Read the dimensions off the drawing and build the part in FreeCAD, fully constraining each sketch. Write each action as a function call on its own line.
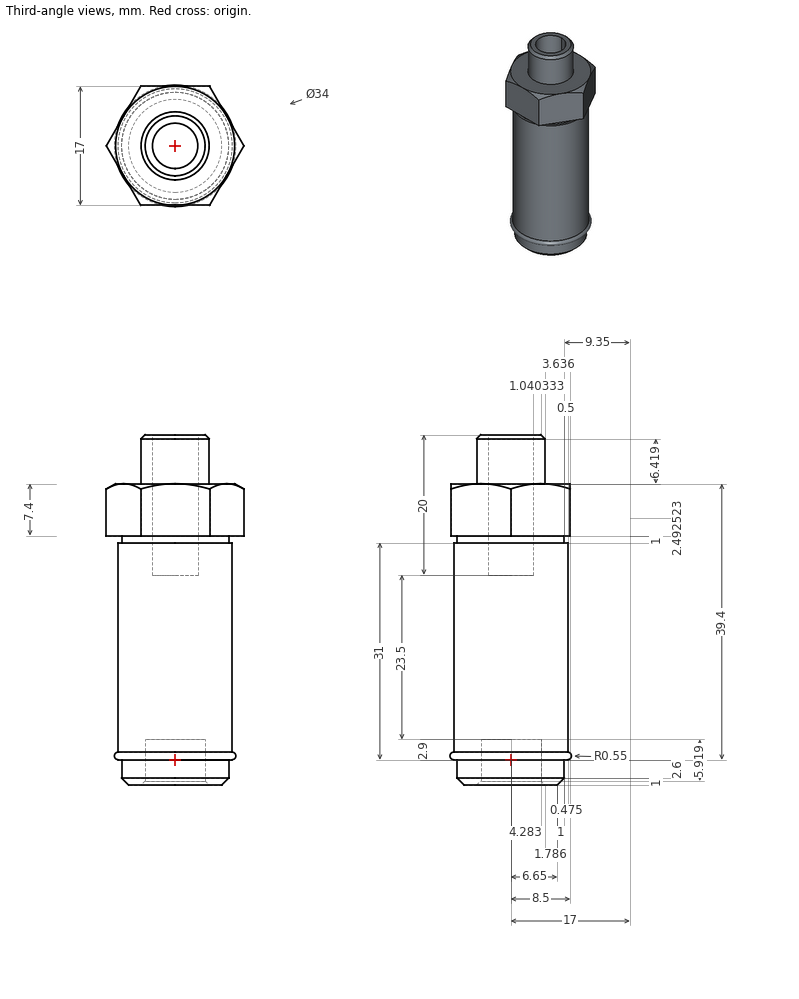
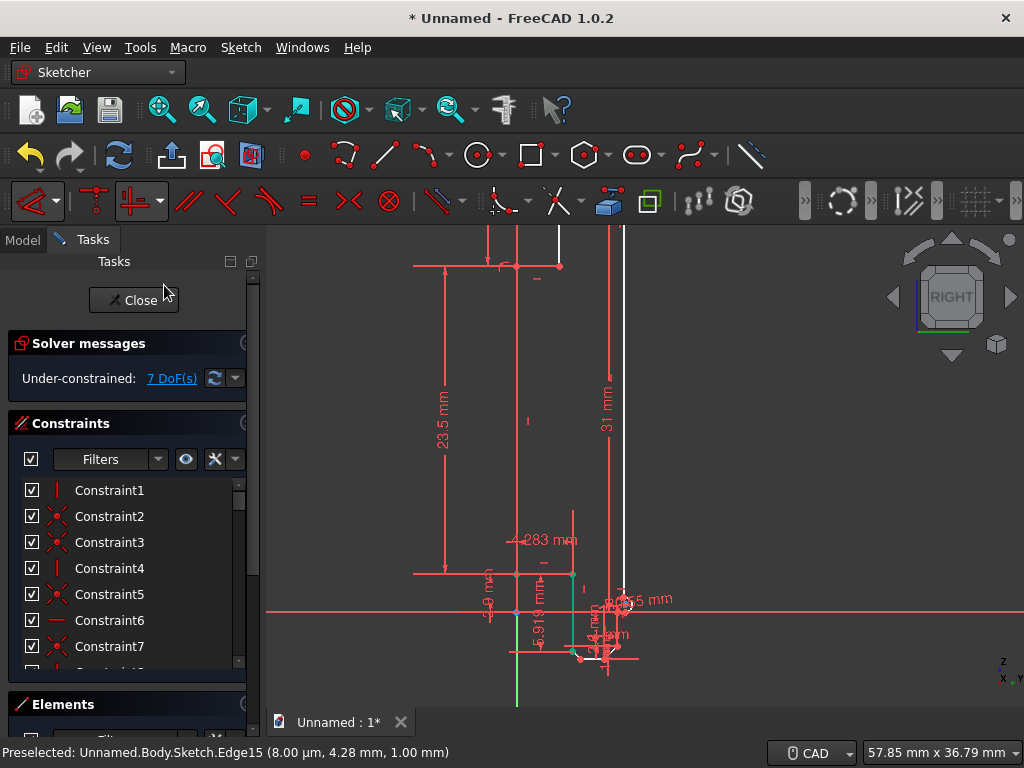
scroll(590, 659, up, 3)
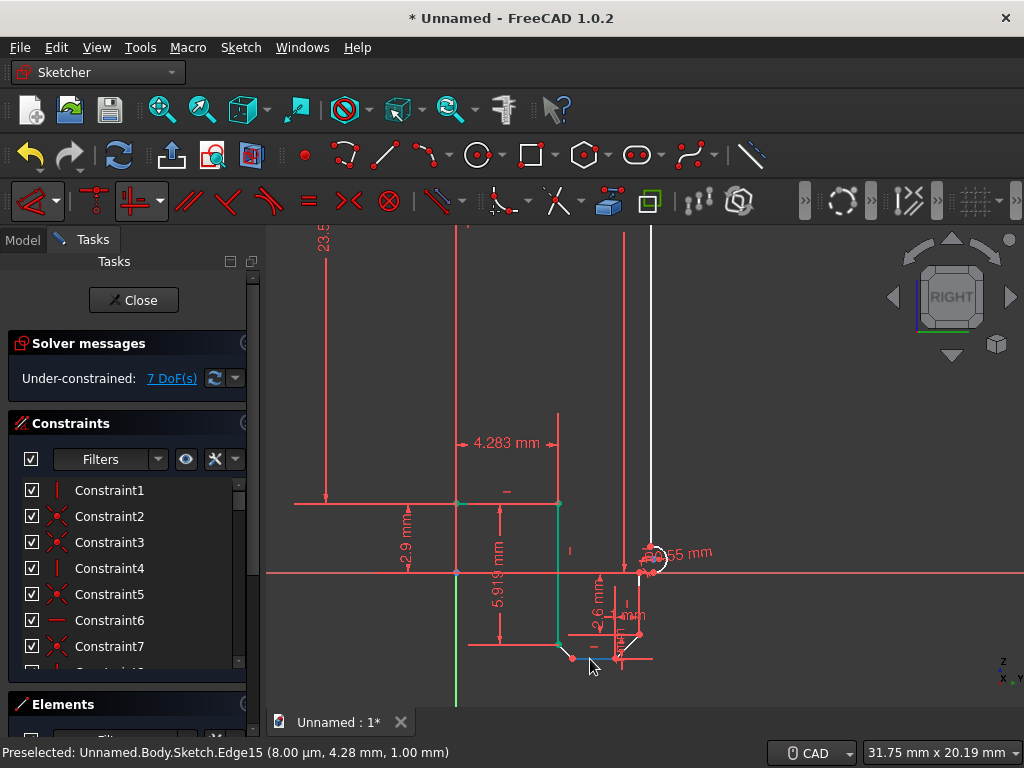
click(590, 659)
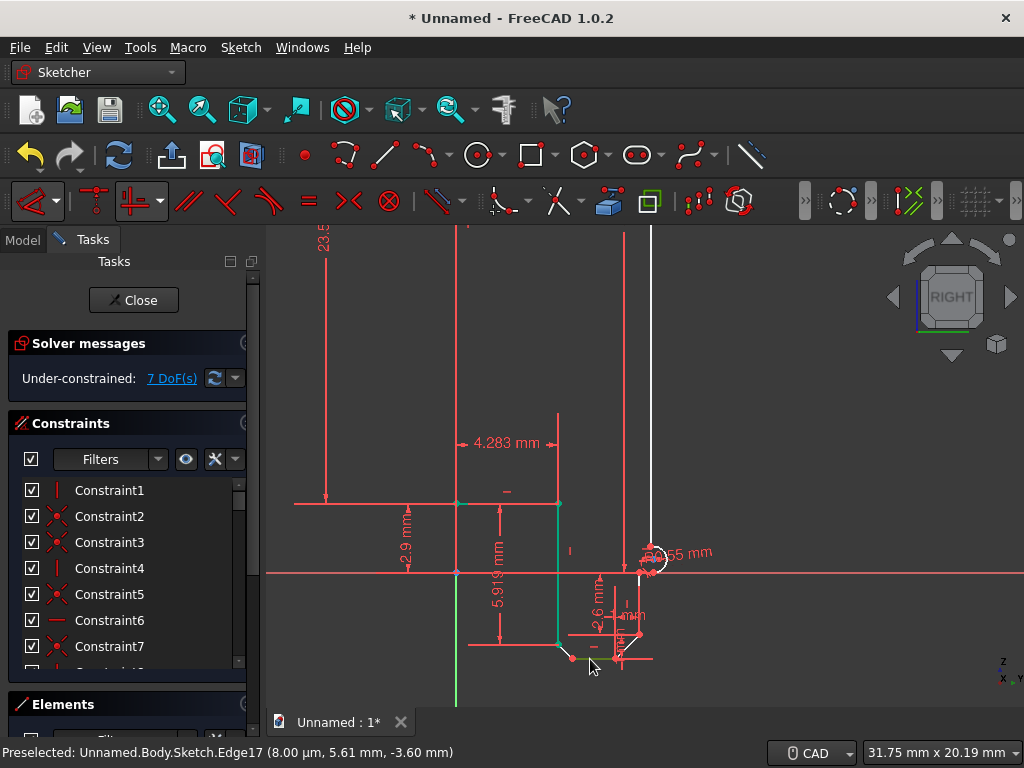
key(l)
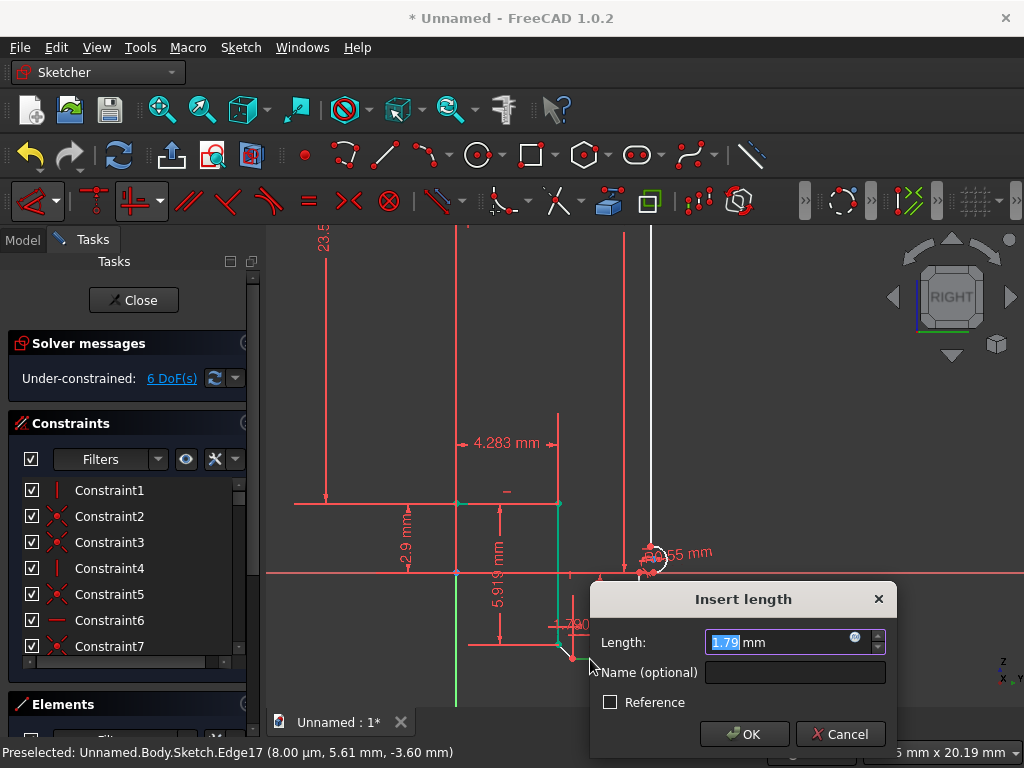
text(1.786)
key(Return)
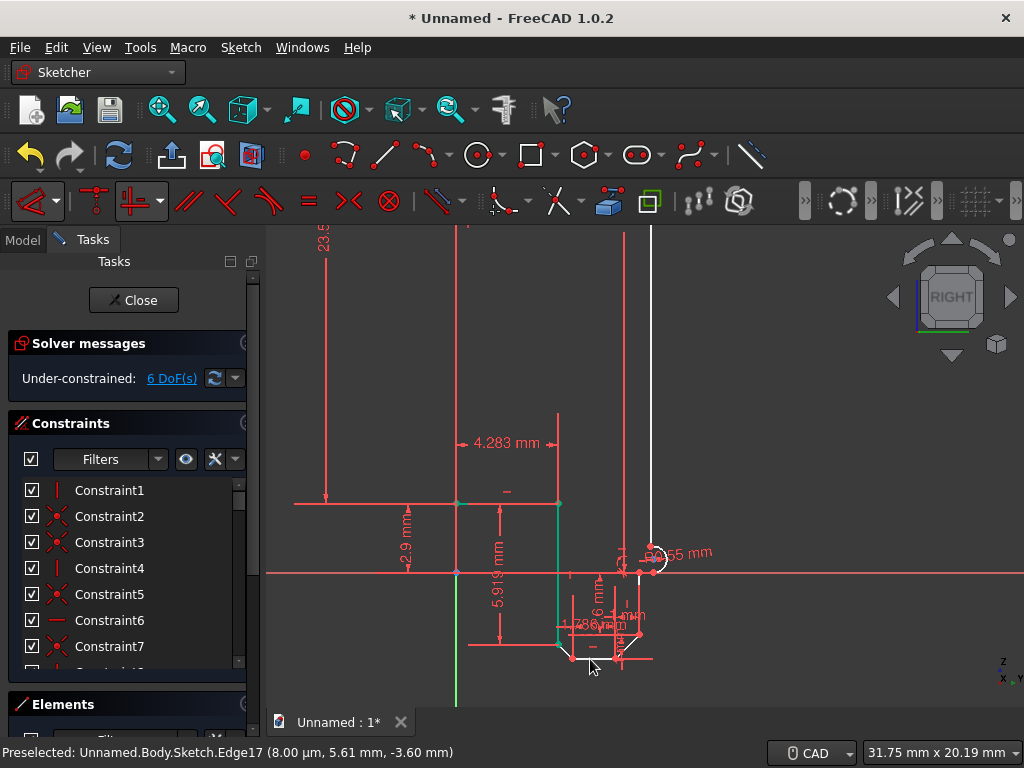
scroll(646, 573, up, 7)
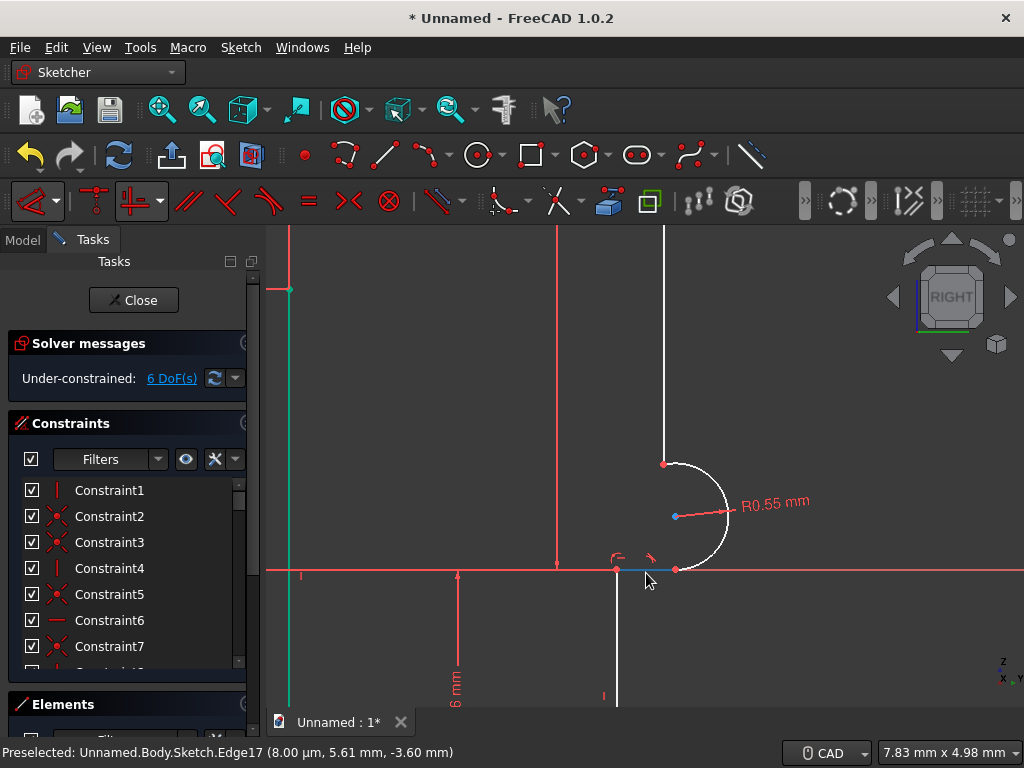
click(646, 570)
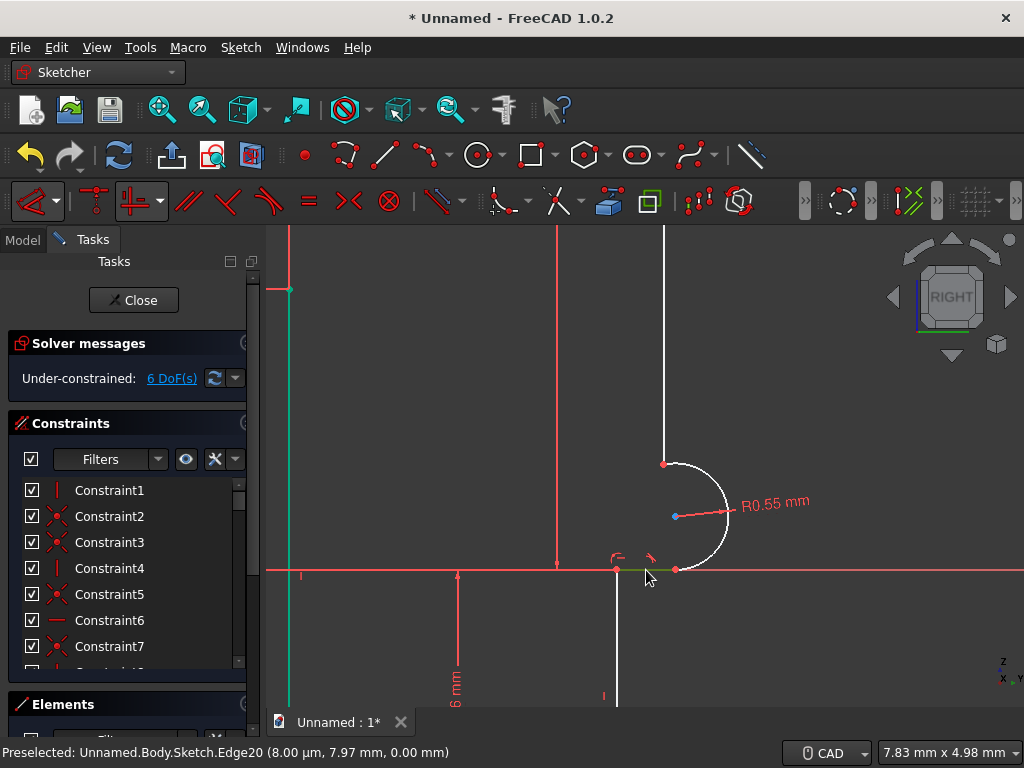
key(l)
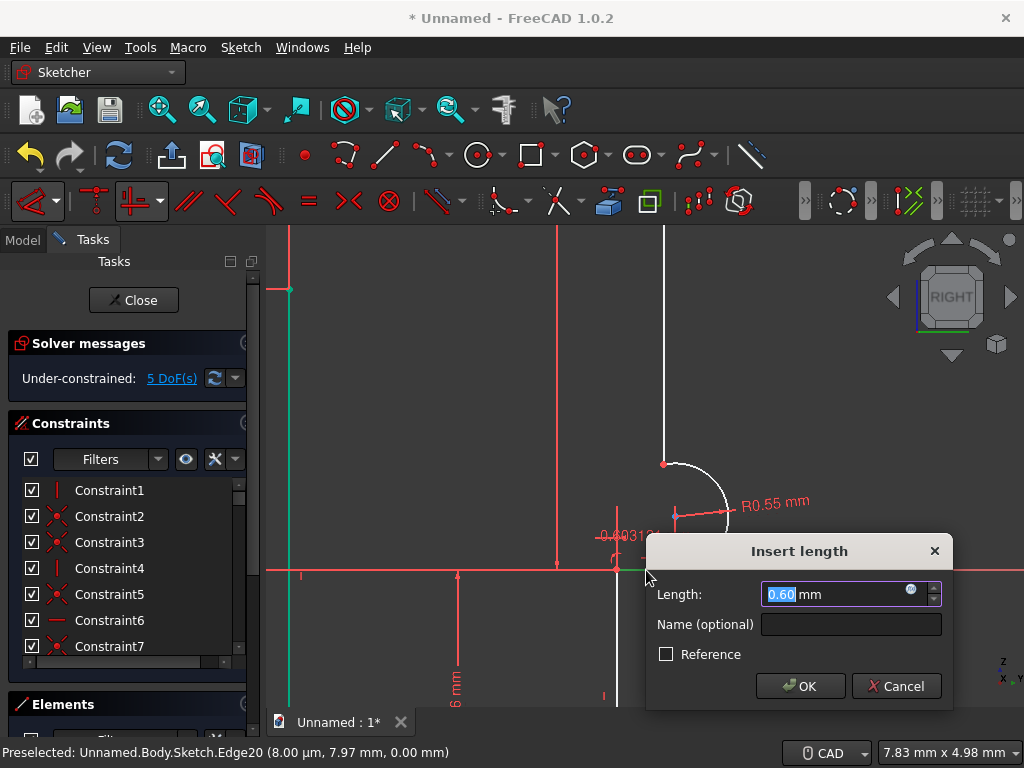
text(0.475)
key(Return)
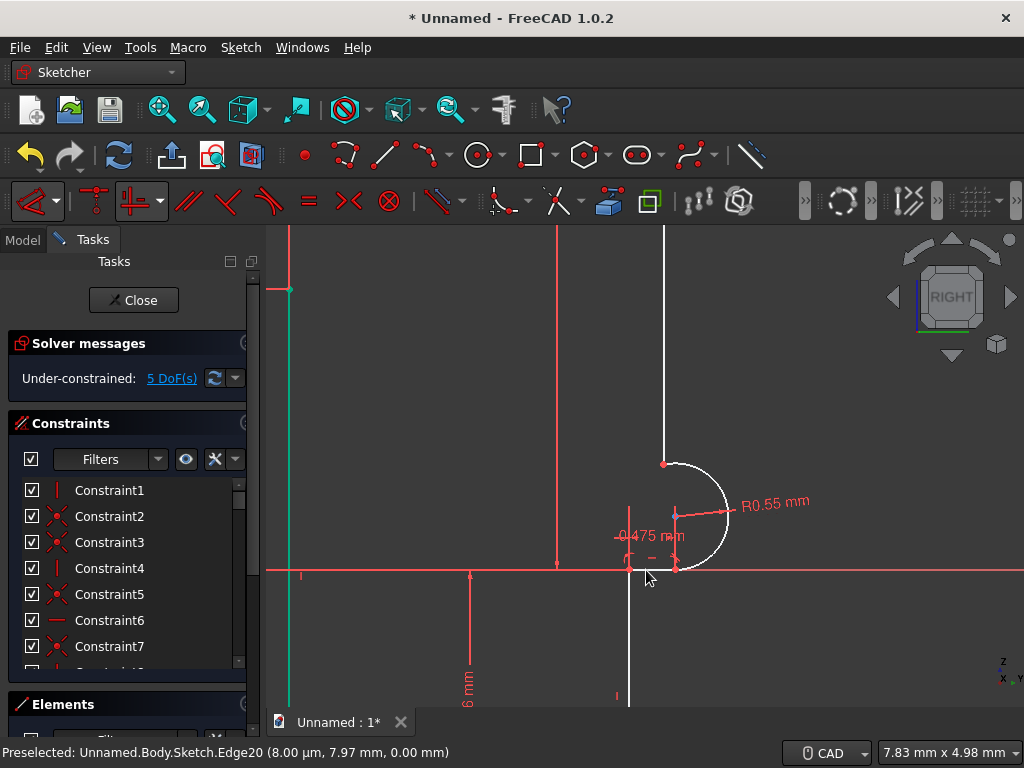
scroll(569, 593, down, 14)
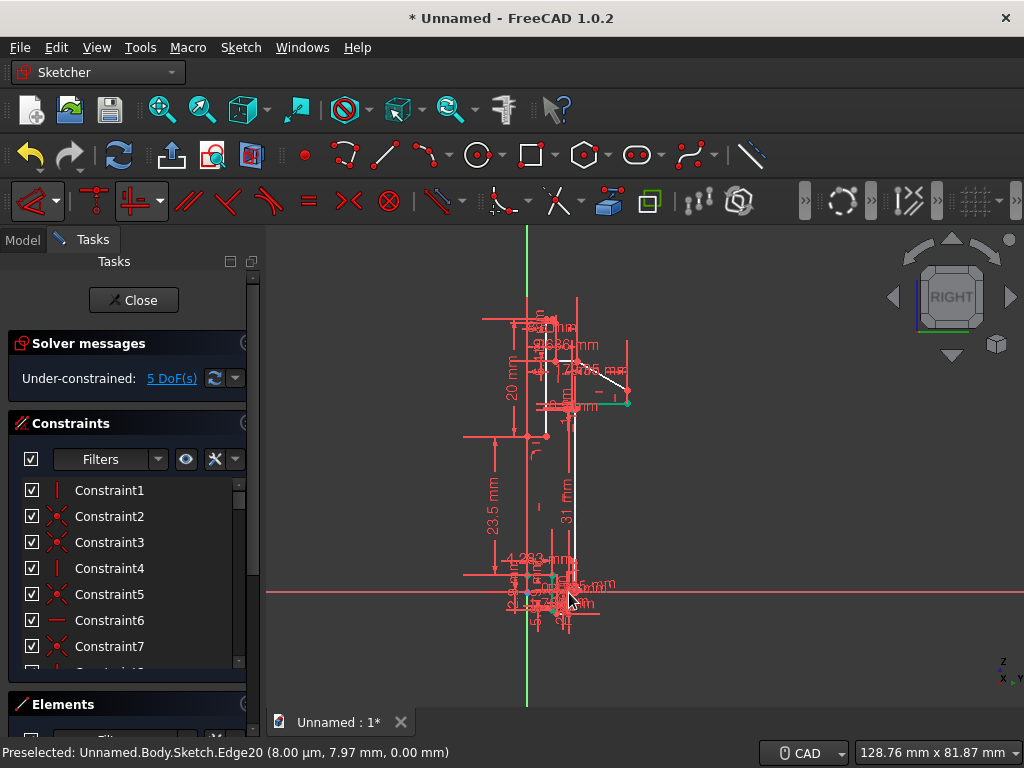
click(577, 361)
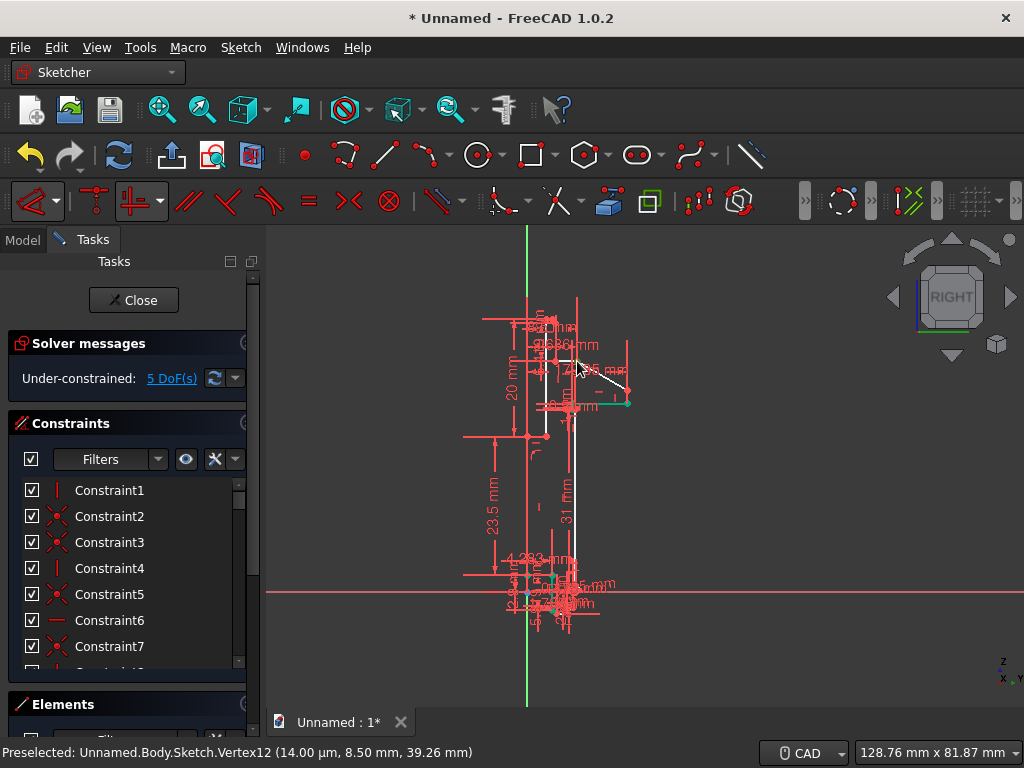
key(i)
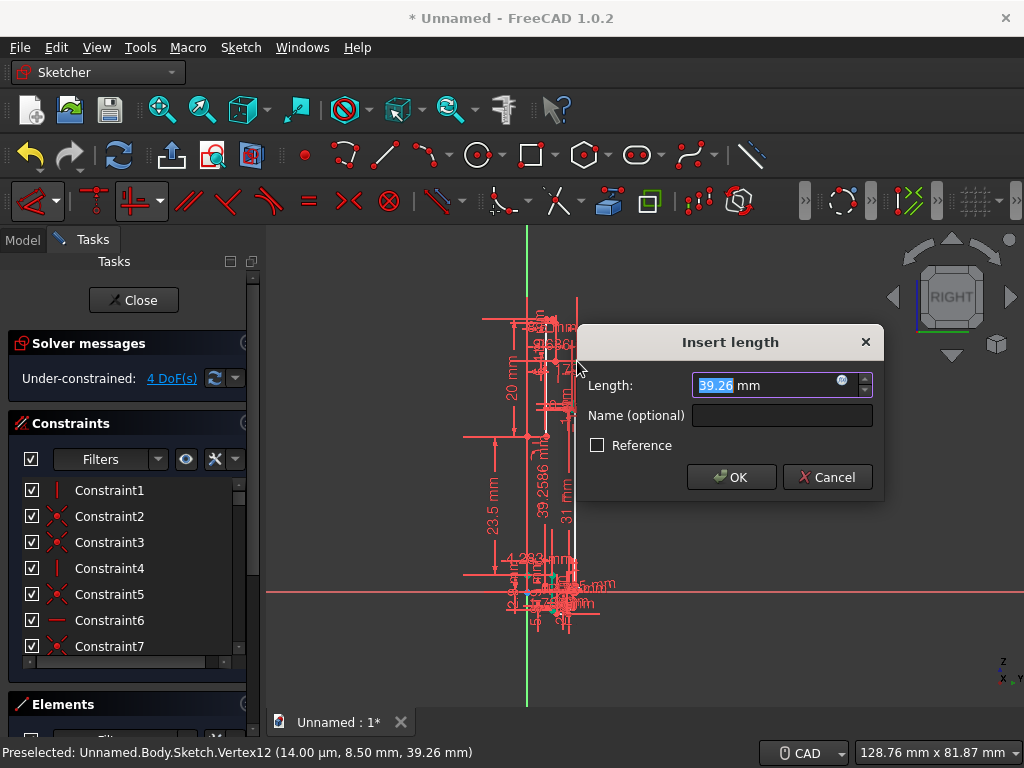
text(39.4)
key(Return)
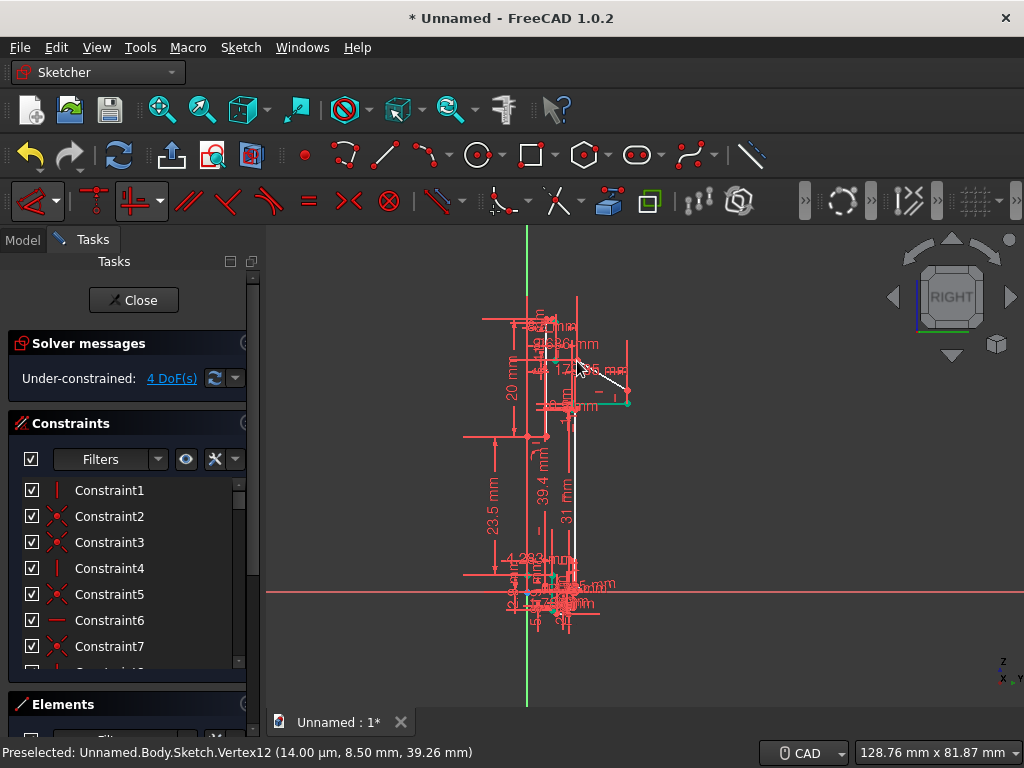
scroll(567, 614, up, 2)